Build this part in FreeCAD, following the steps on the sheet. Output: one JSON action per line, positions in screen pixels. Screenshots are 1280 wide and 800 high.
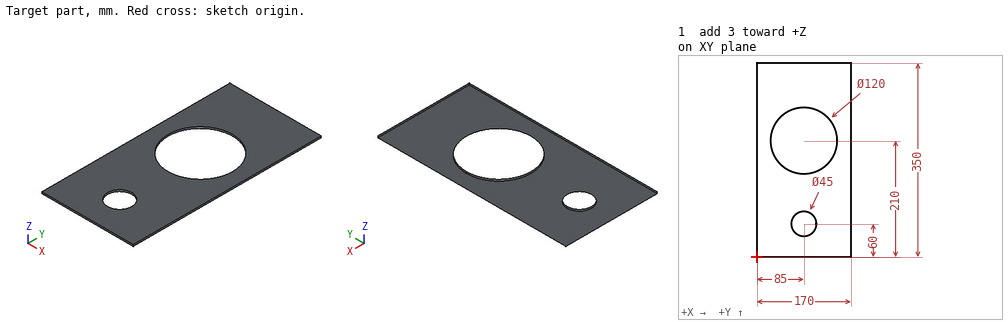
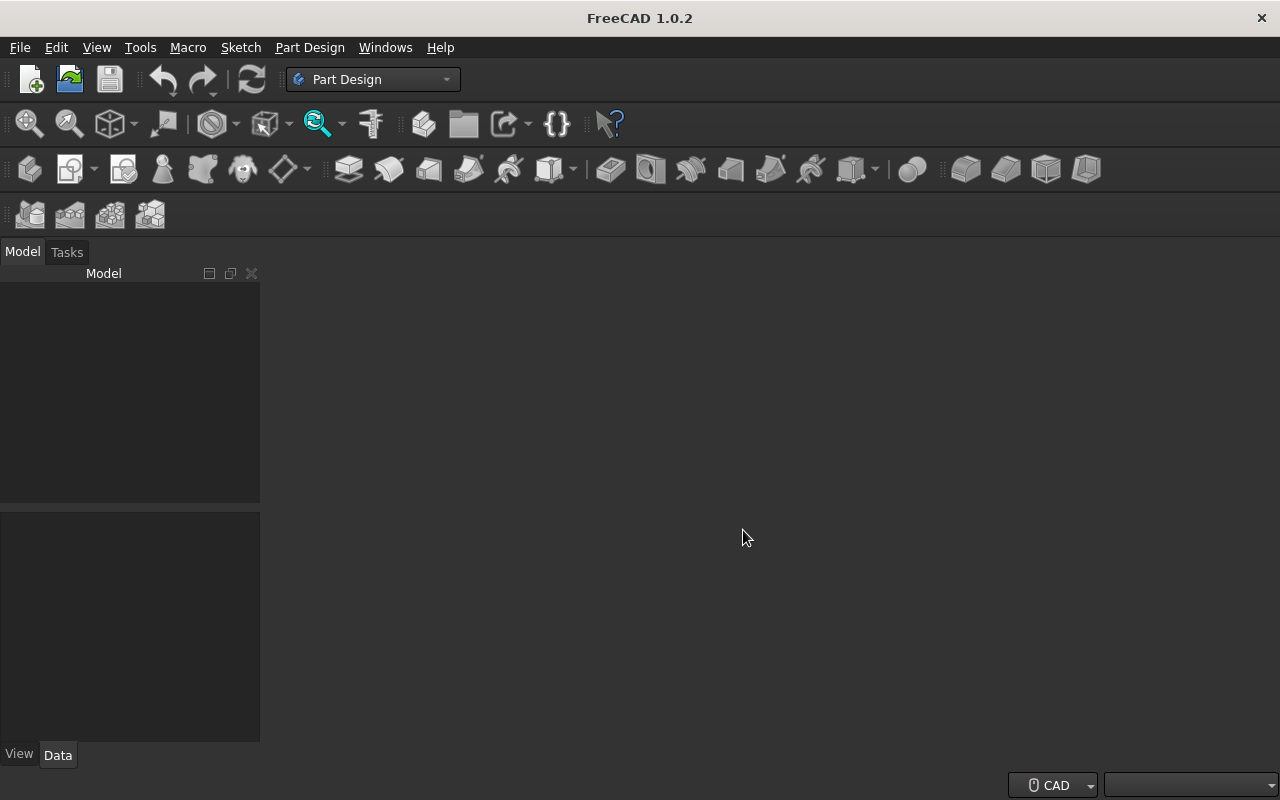
{"action": "left_click", "coordinate": [30, 80]}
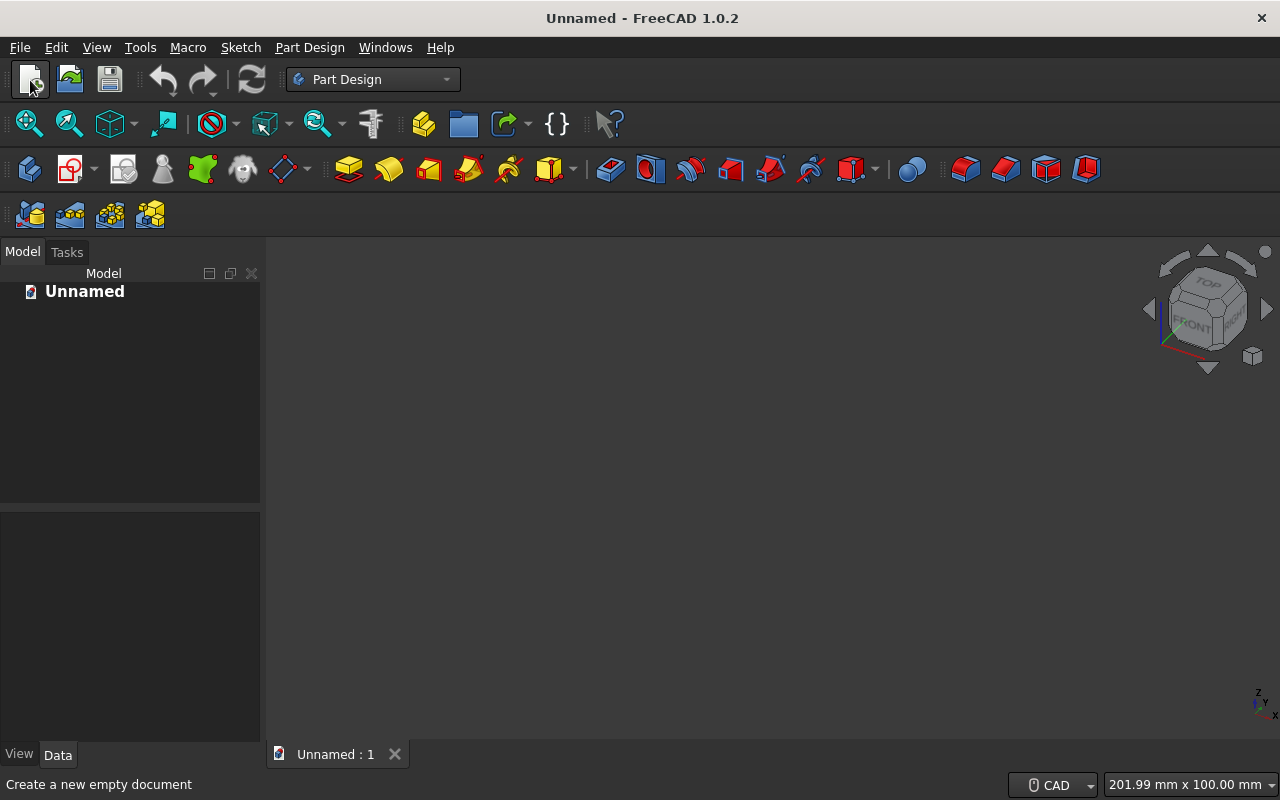
{"action": "left_click", "coordinate": [70, 170]}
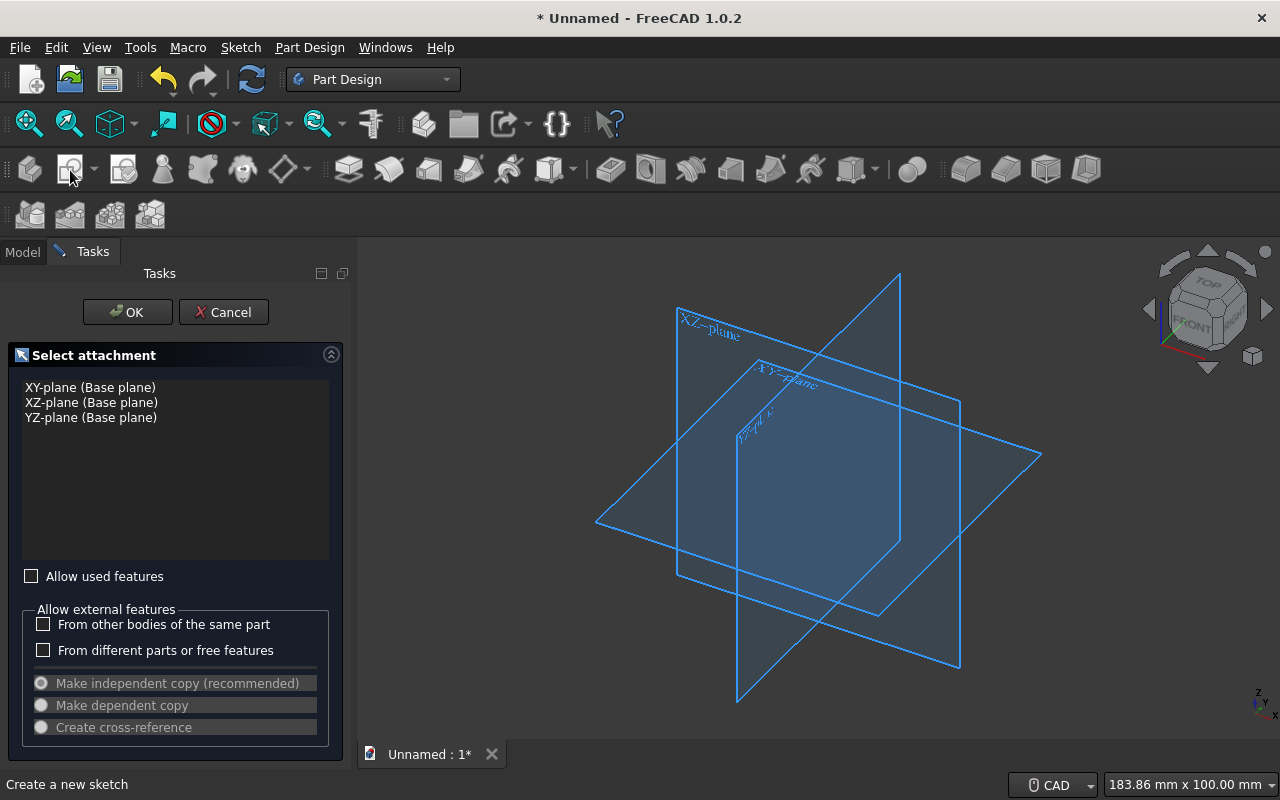
{"action": "left_click", "coordinate": [82, 388]}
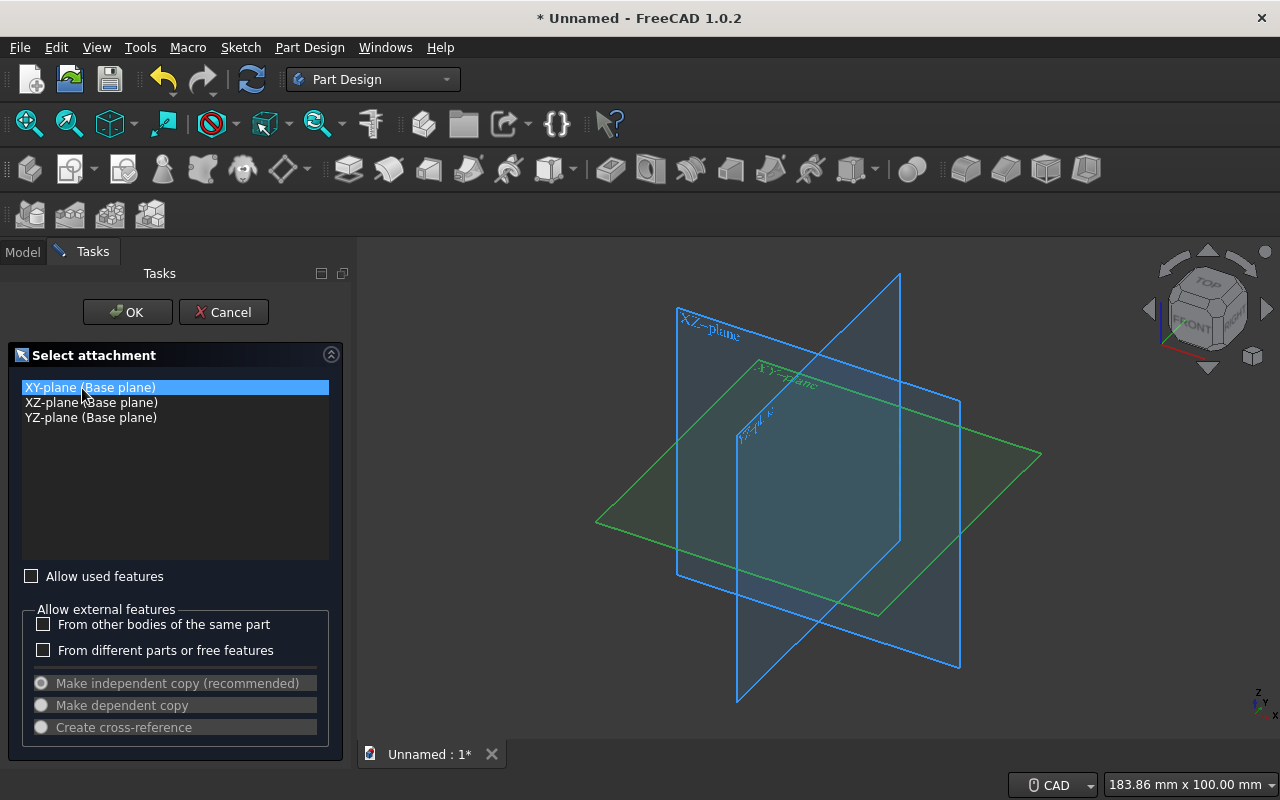
{"action": "left_click", "coordinate": [128, 312]}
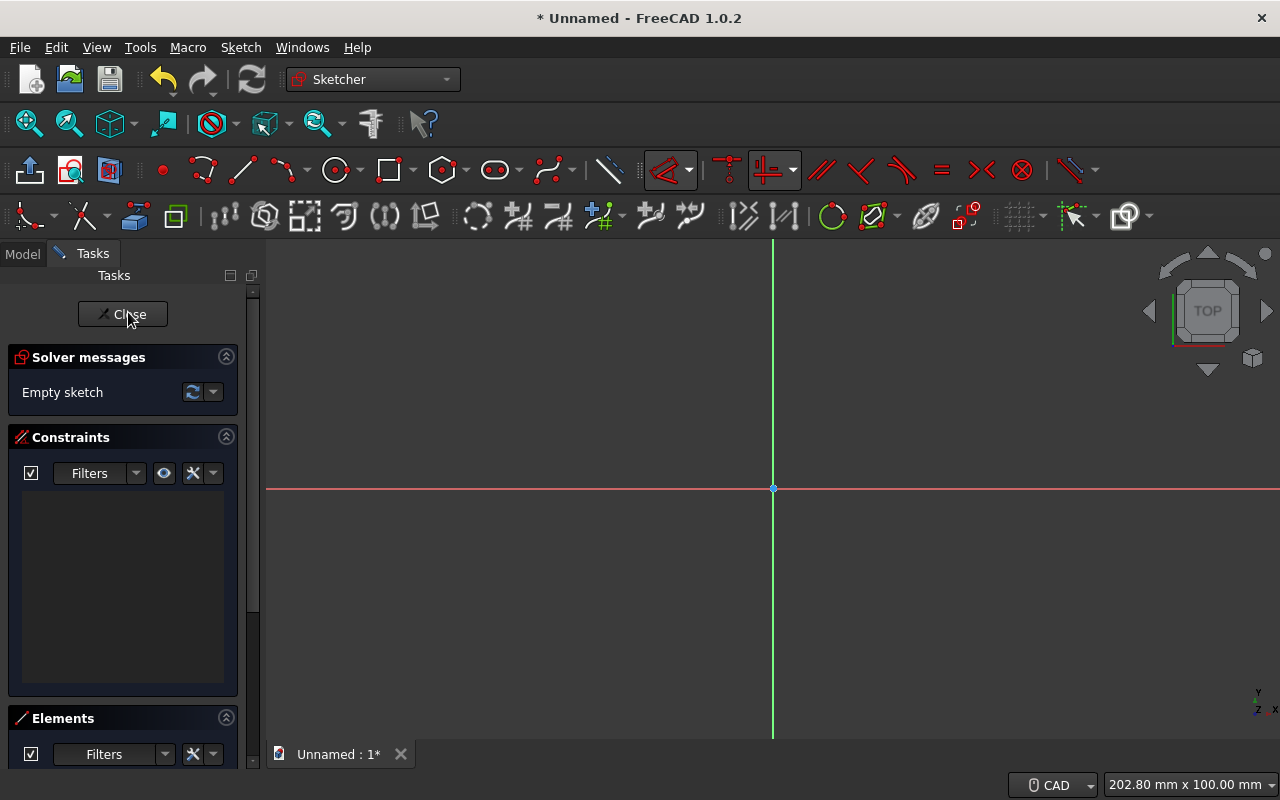
{"action": "scroll", "coordinate": [607, 662], "scroll_direction": "down", "scroll_amount": 9}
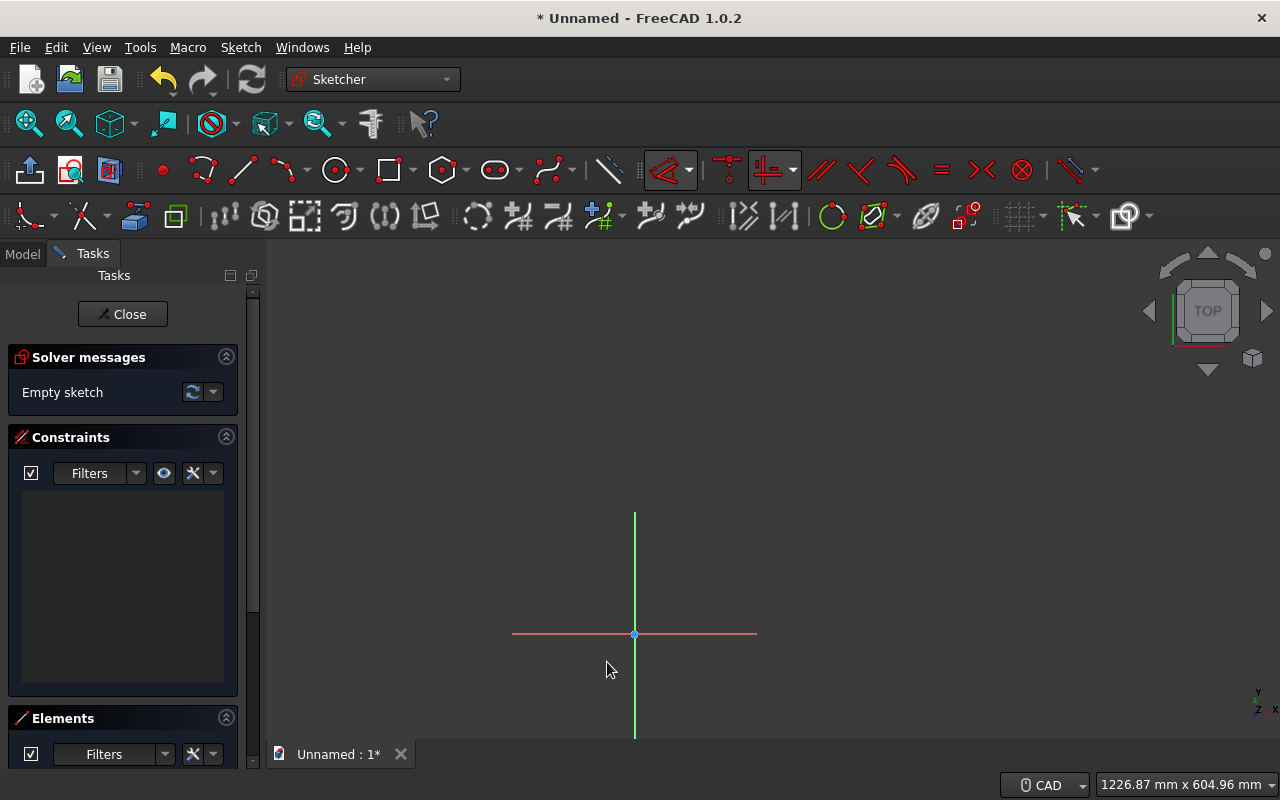
{"action": "left_click", "coordinate": [390, 170]}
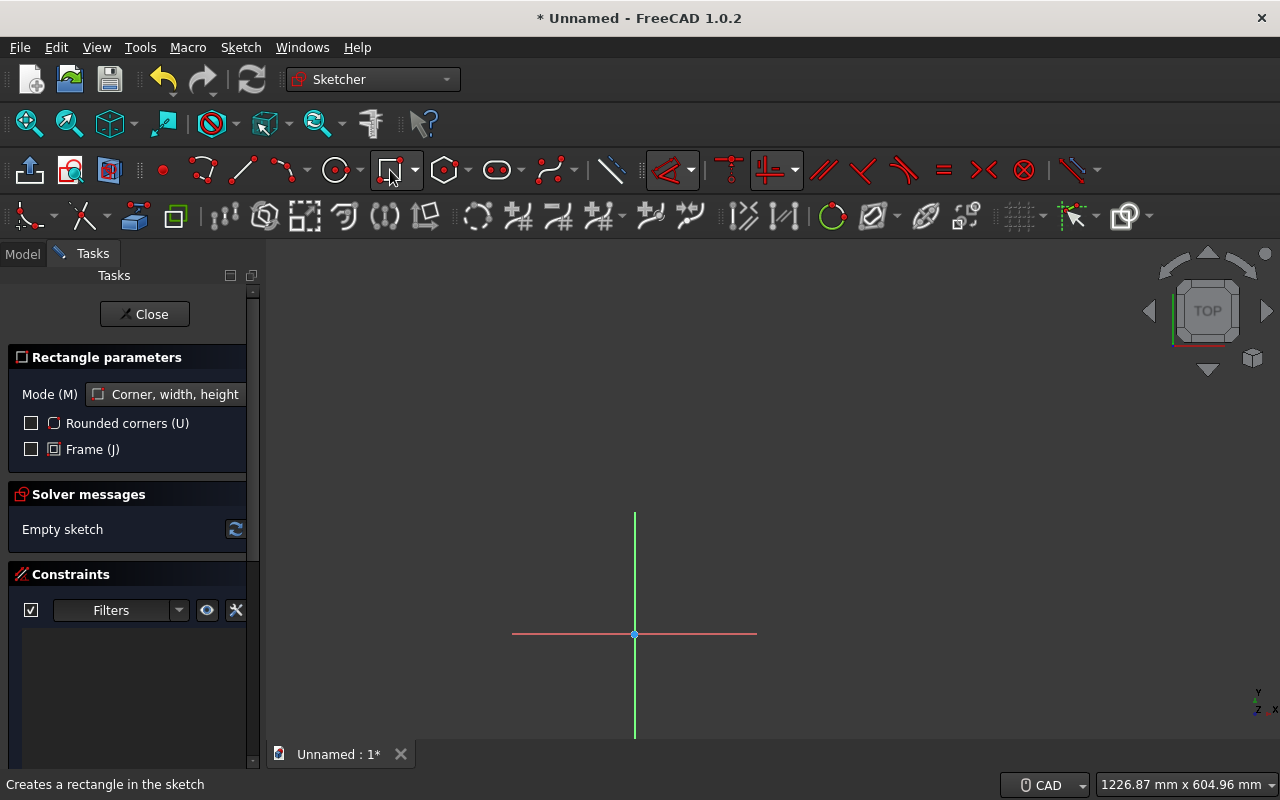
{"action": "left_click", "coordinate": [635, 634]}
{"action": "mouse_move", "coordinate": [775, 345]}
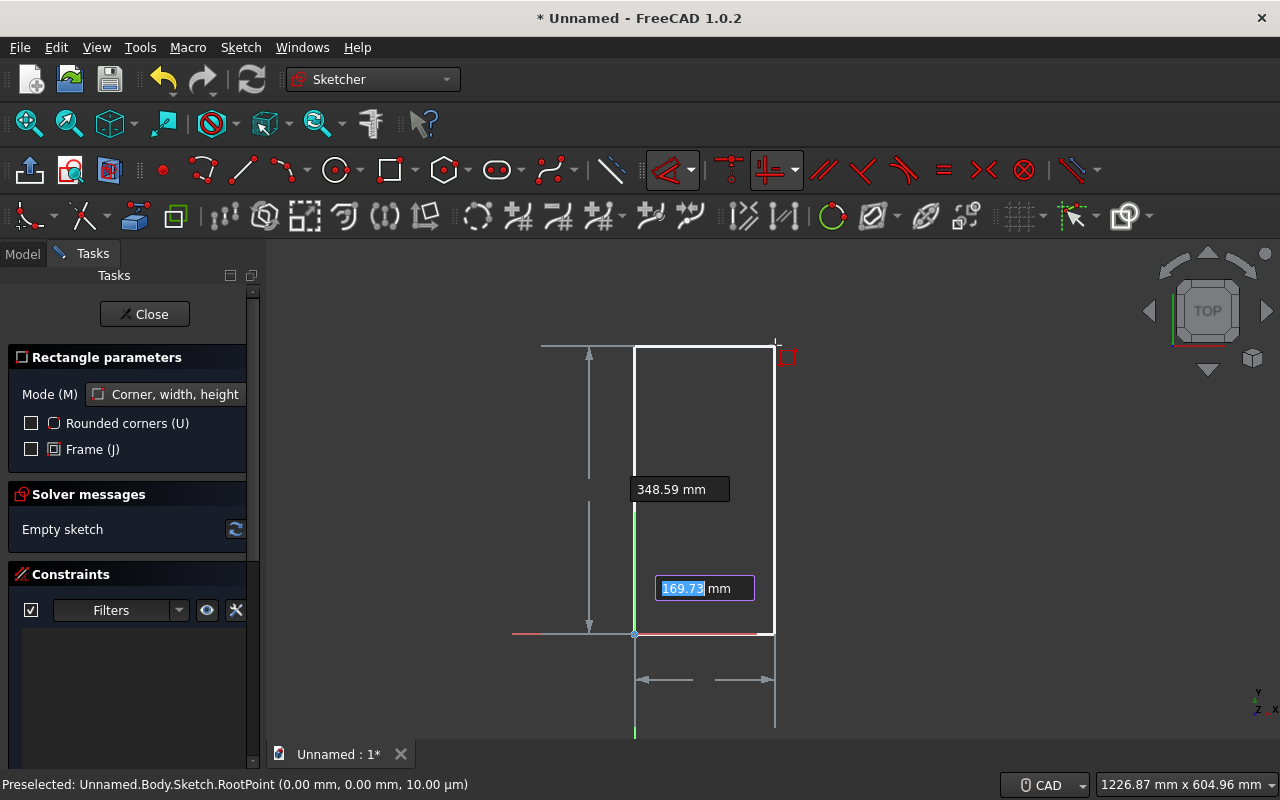
{"action": "type", "text": "170"}
{"action": "key", "text": "Tab"}
{"action": "type", "text": "350"}
{"action": "key", "text": "Return"}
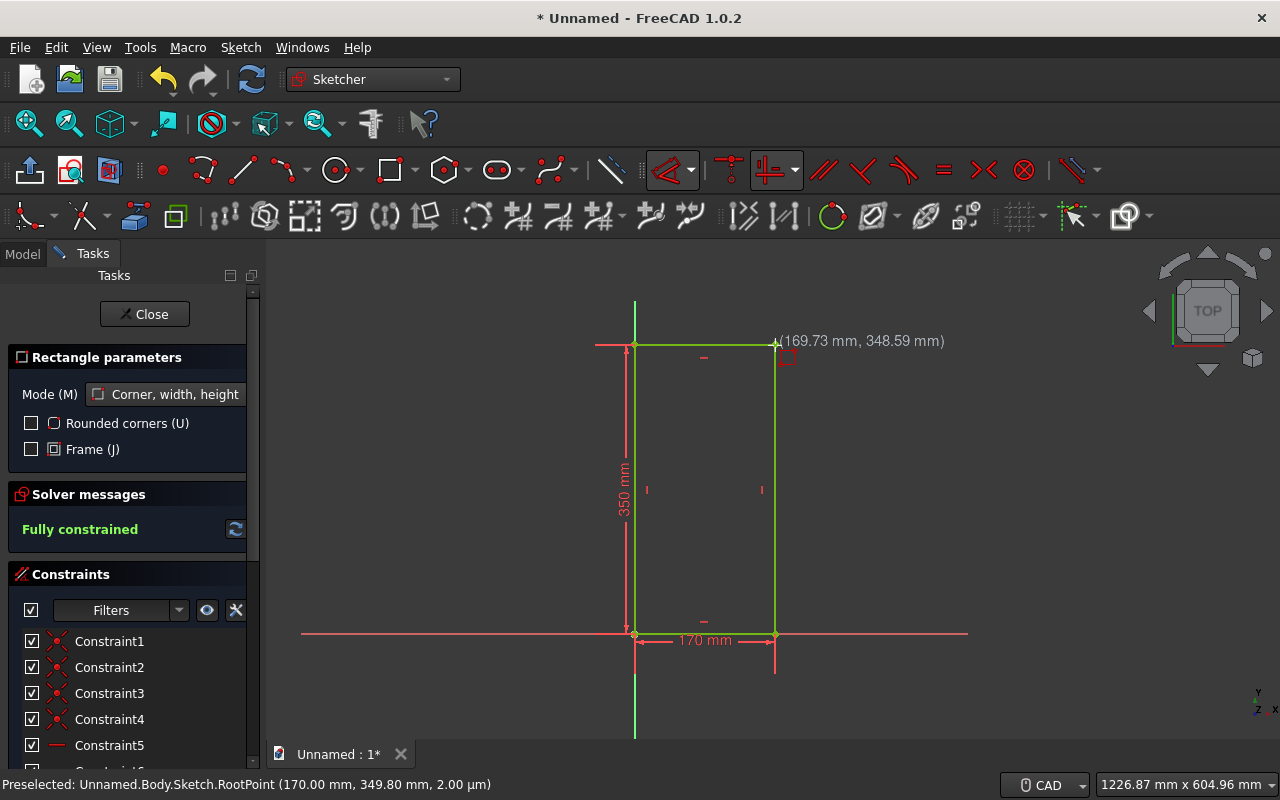
{"action": "left_click", "coordinate": [336, 170]}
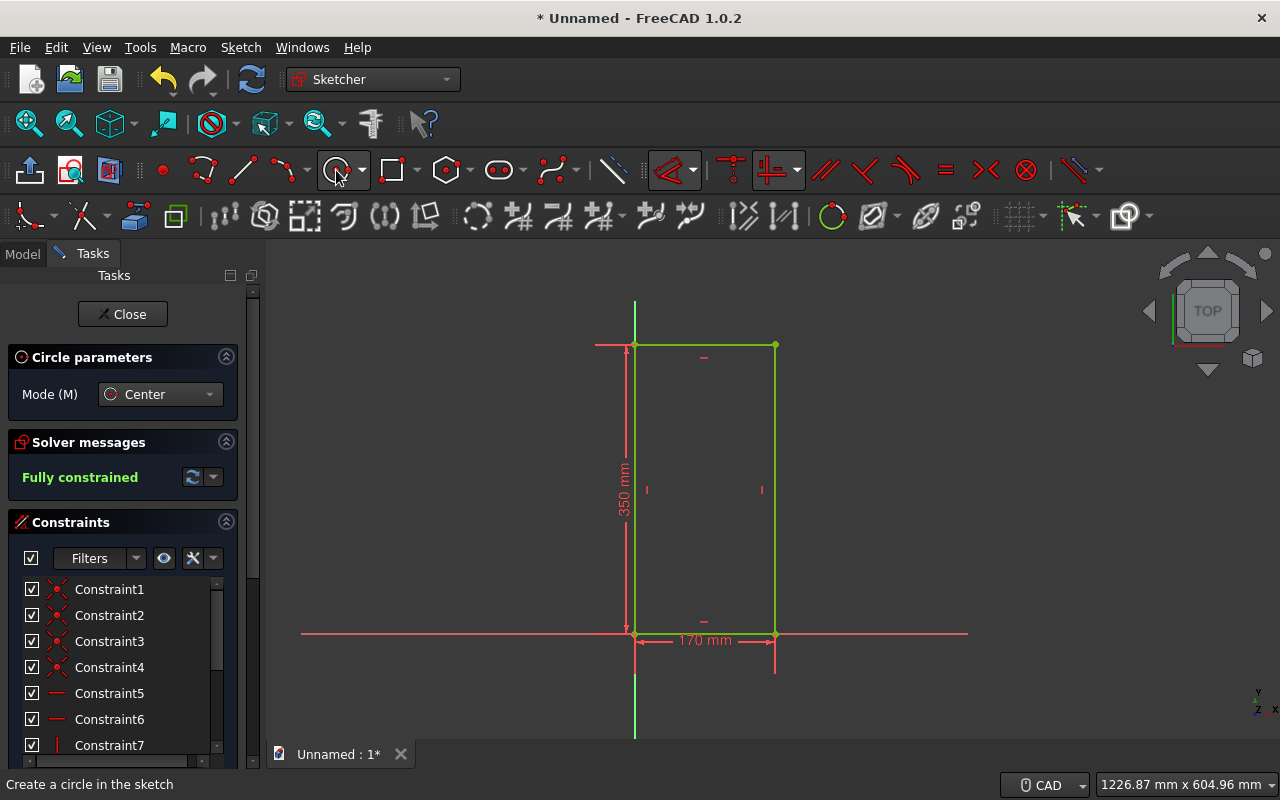
{"action": "left_click", "coordinate": [705, 585]}
{"action": "mouse_move", "coordinate": [718, 571]}